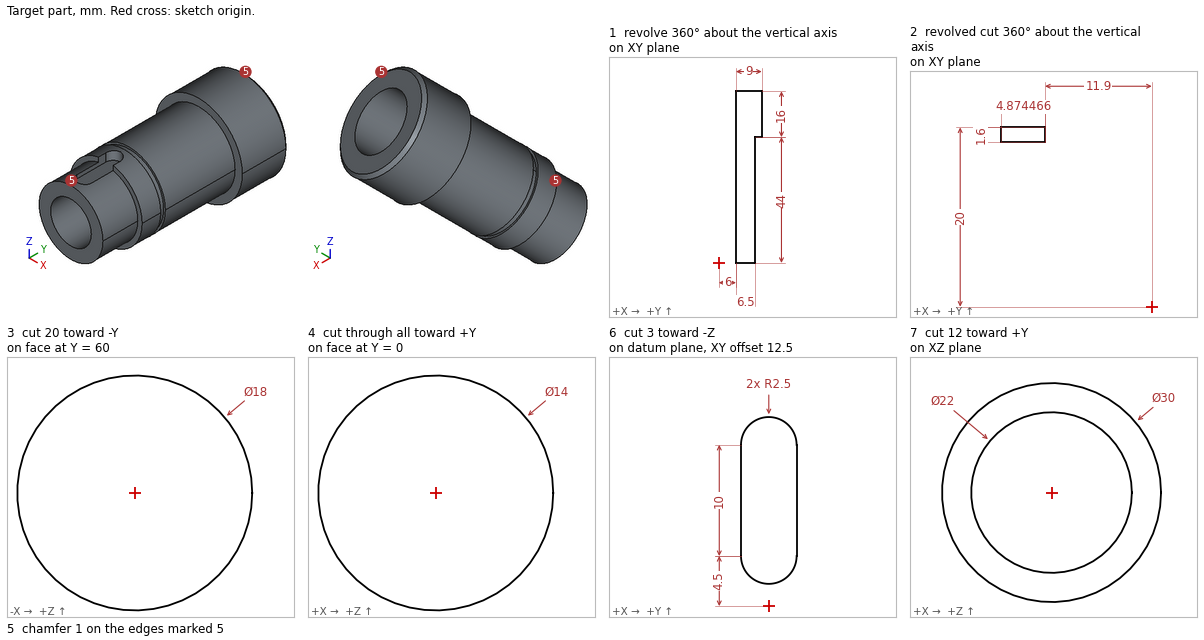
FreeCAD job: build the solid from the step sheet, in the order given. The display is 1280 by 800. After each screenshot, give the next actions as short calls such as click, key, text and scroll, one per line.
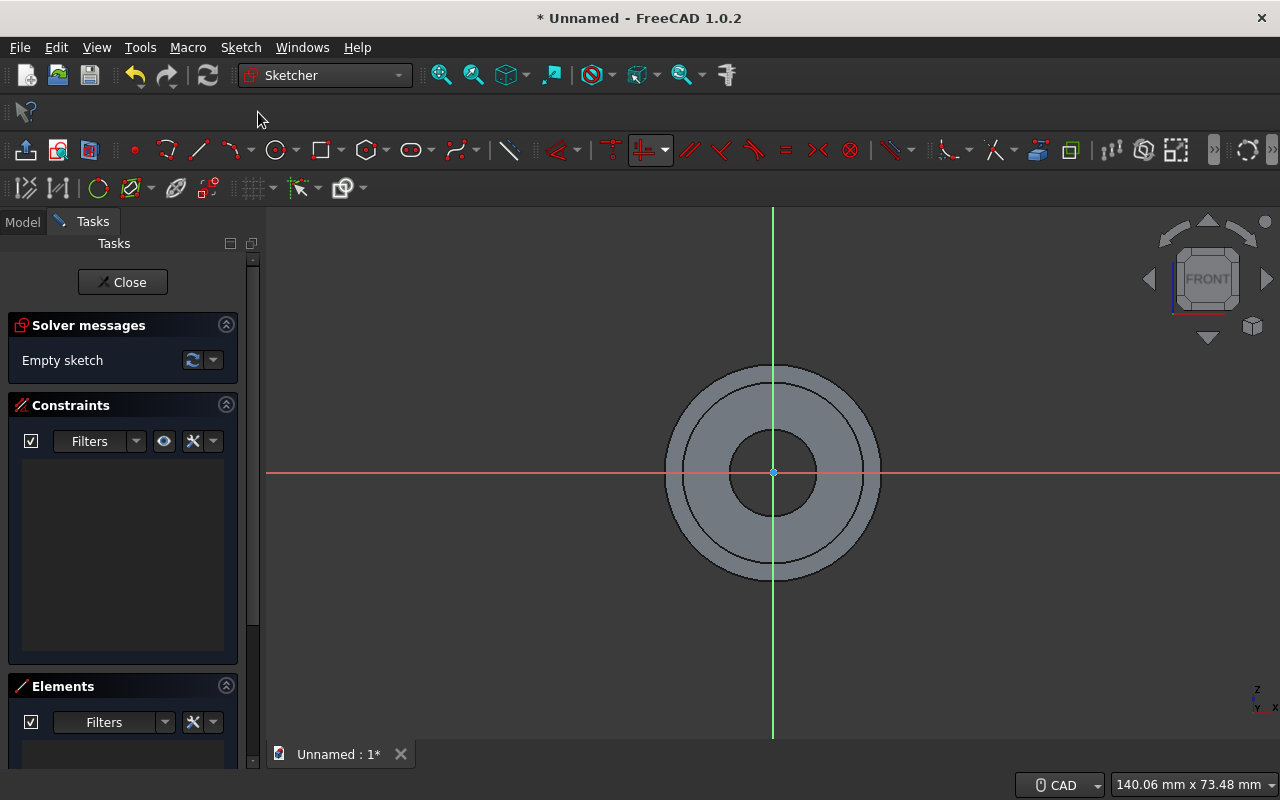
scroll(803, 473, up, 6)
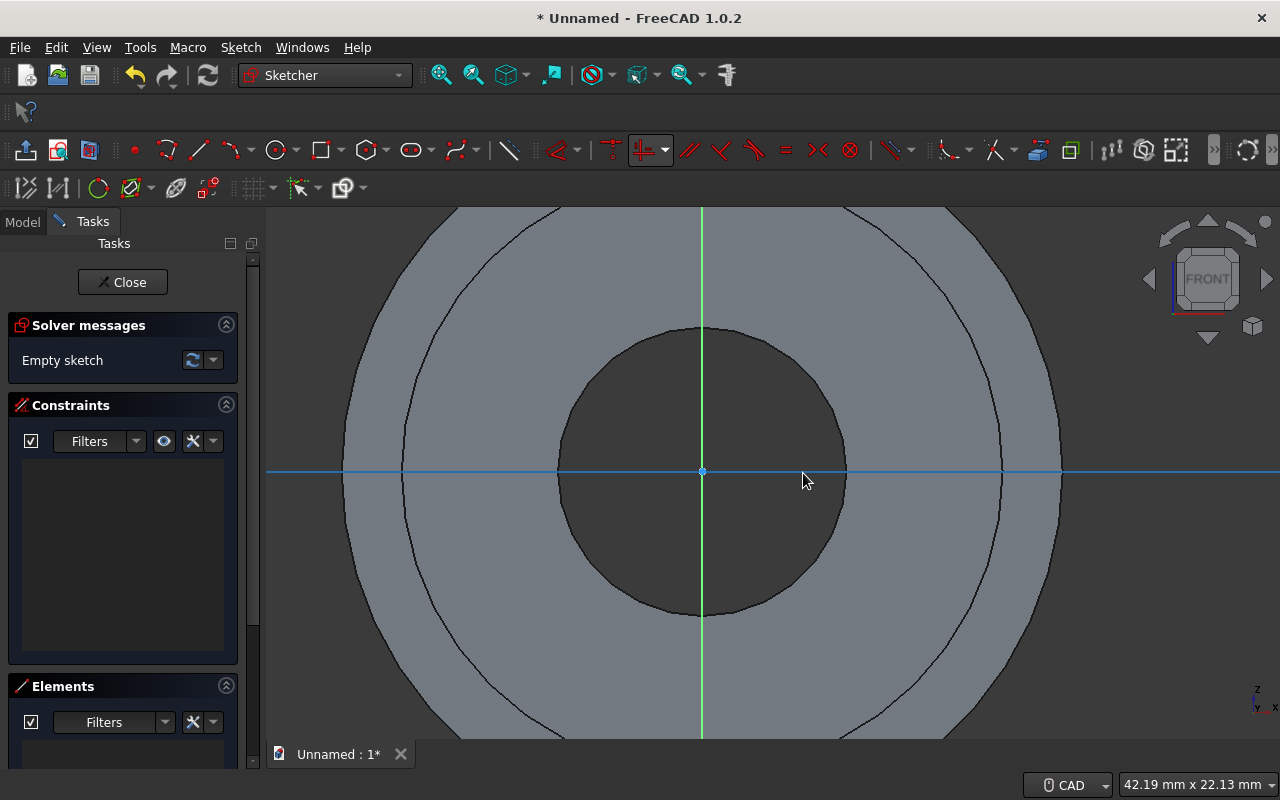
click(276, 150)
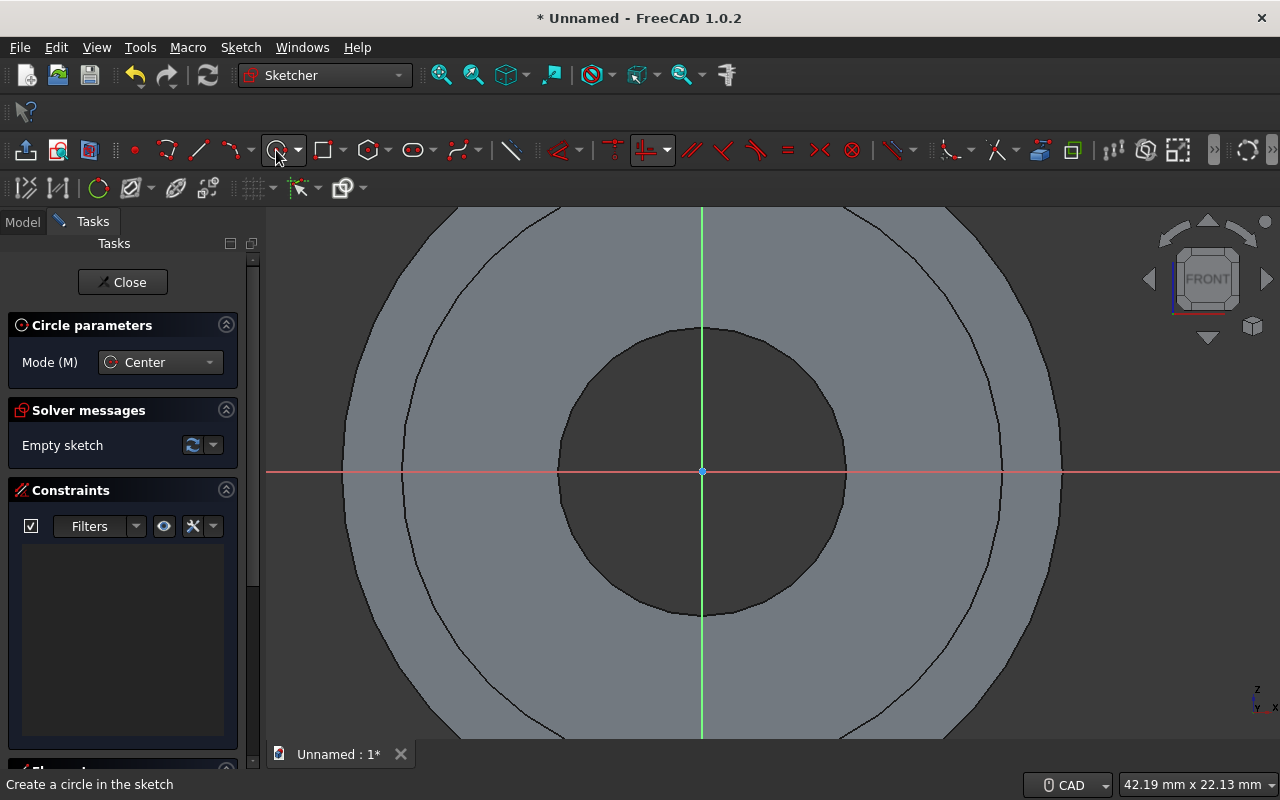
click(702, 472)
move(821, 353)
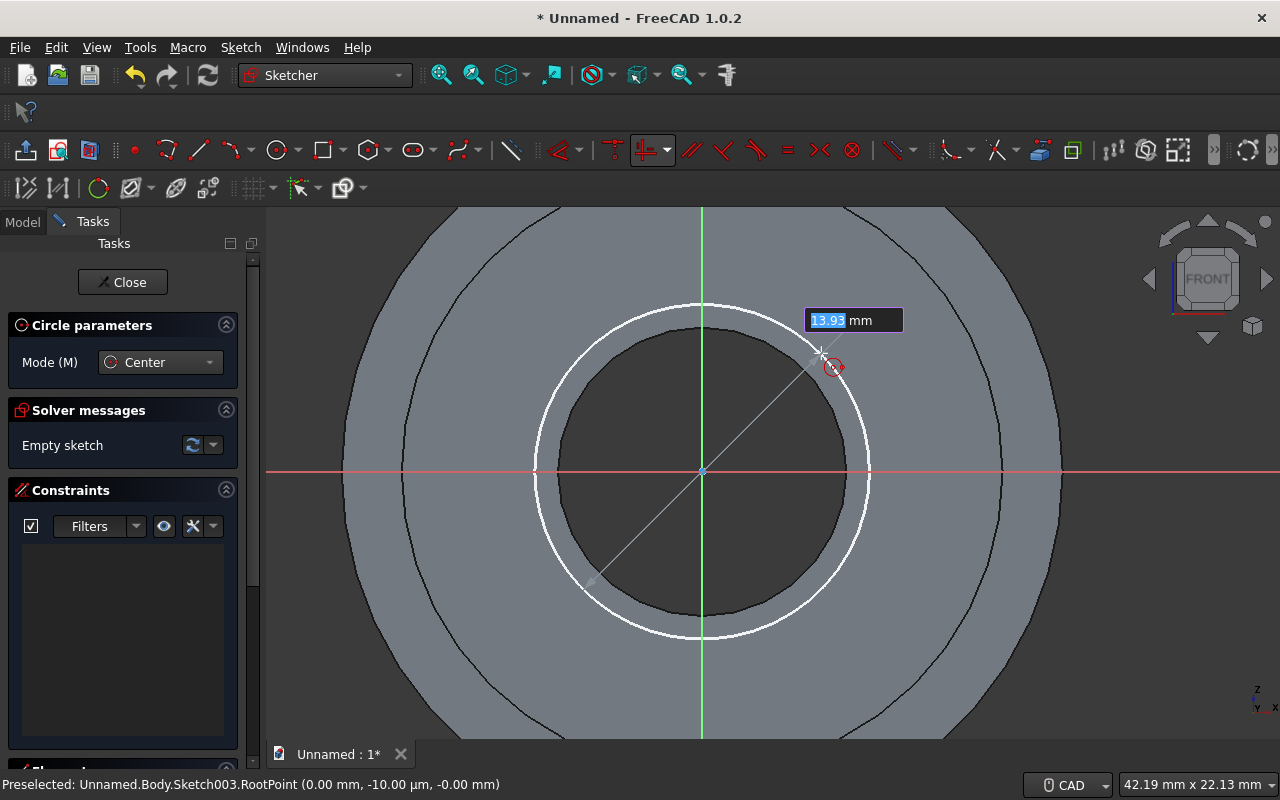
text(14)
key(Return)
key(Escape)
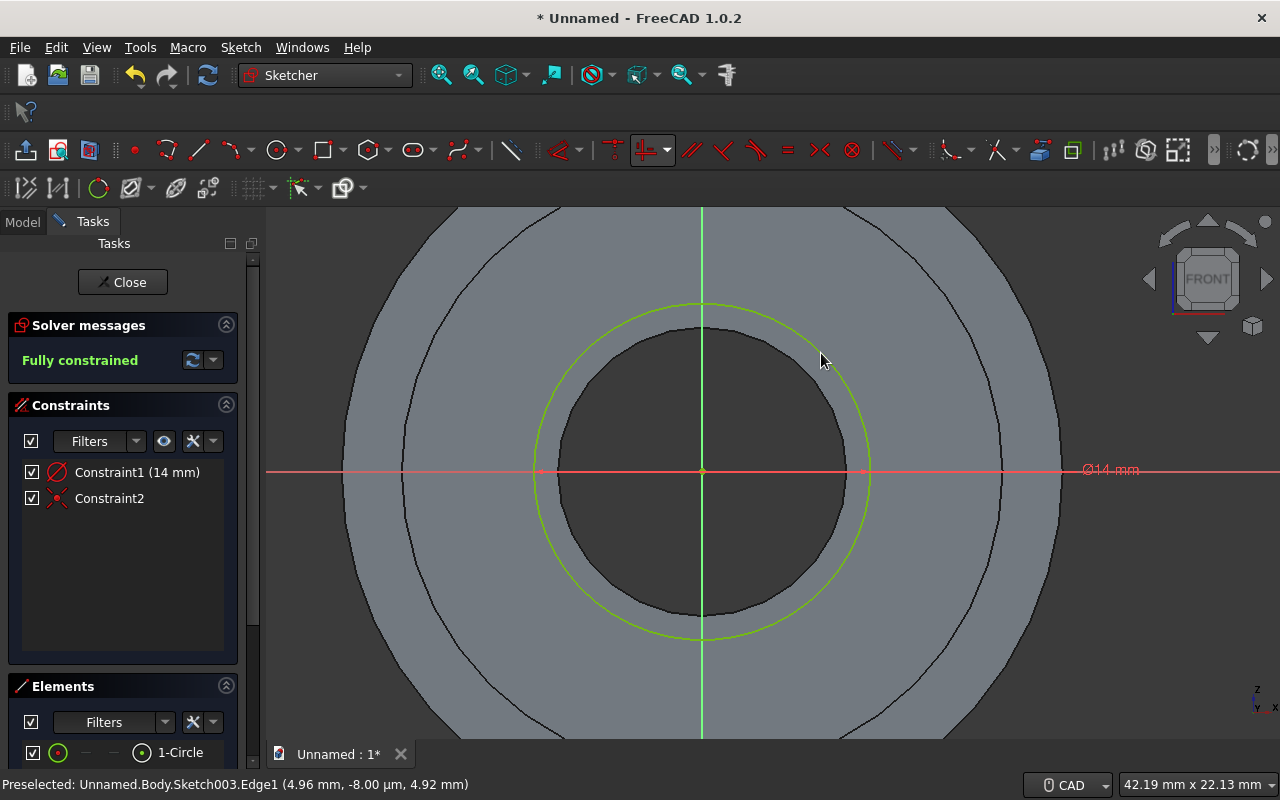
click(123, 282)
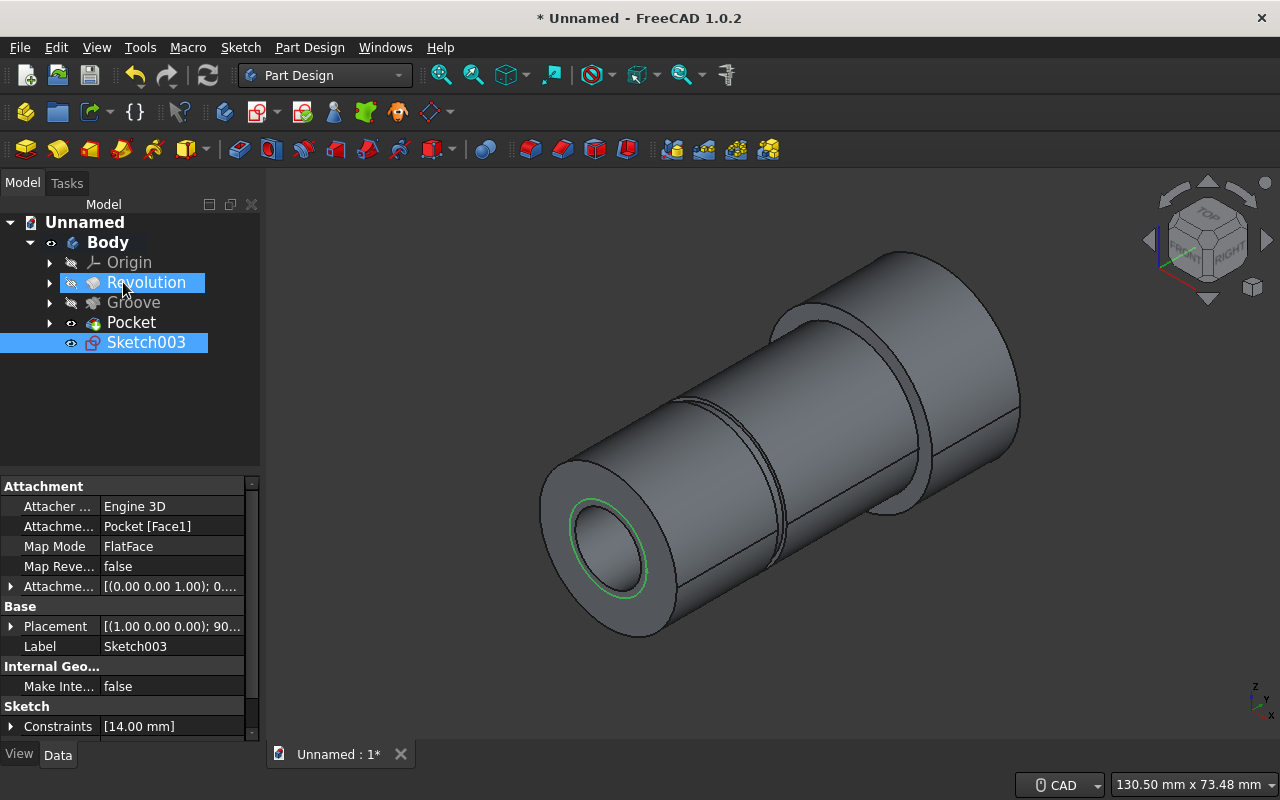
click(240, 150)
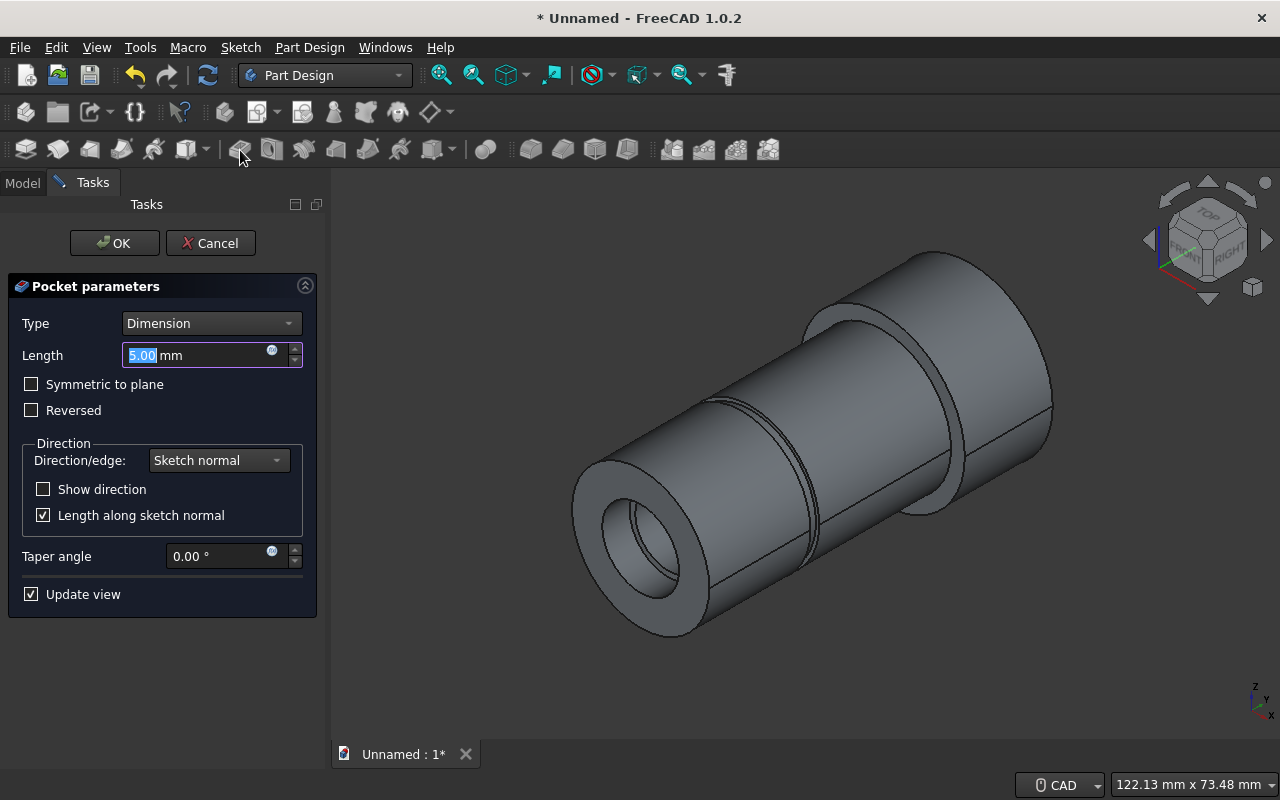
click(212, 324)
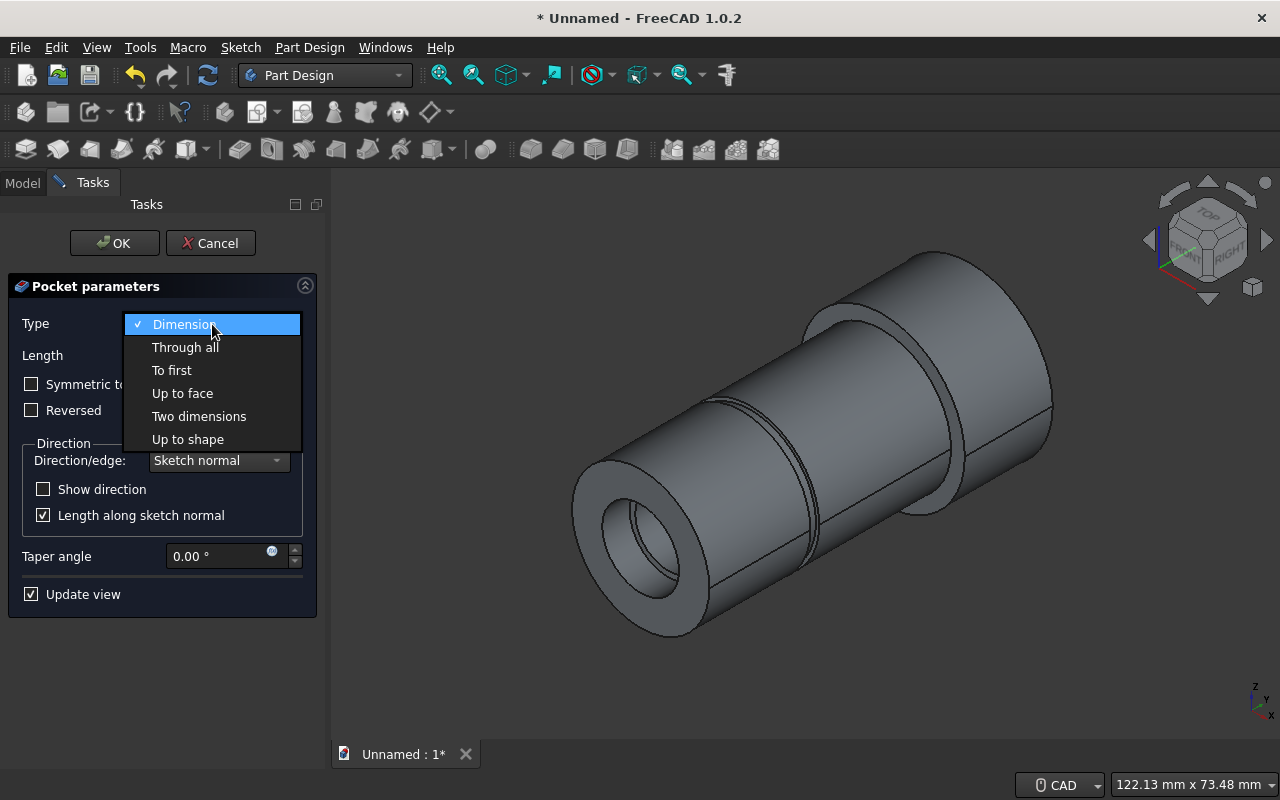
click(212, 348)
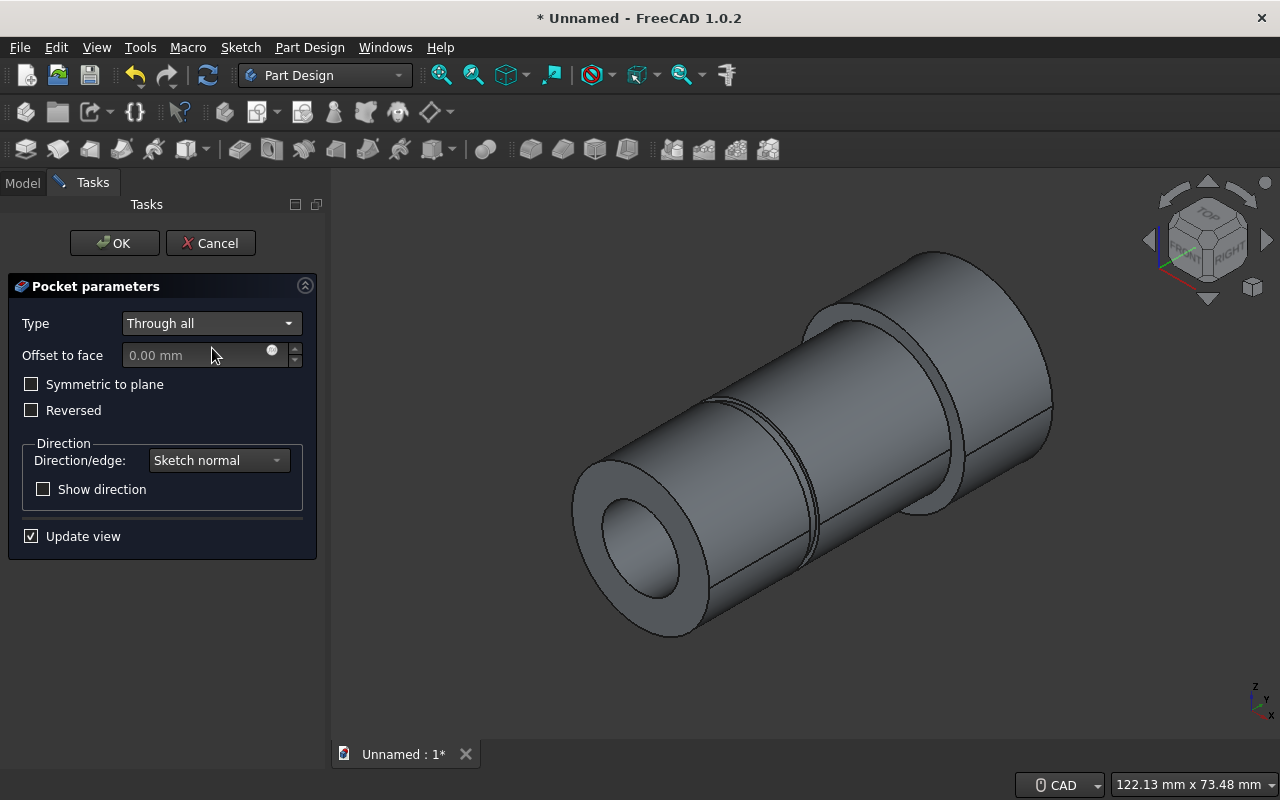
click(115, 243)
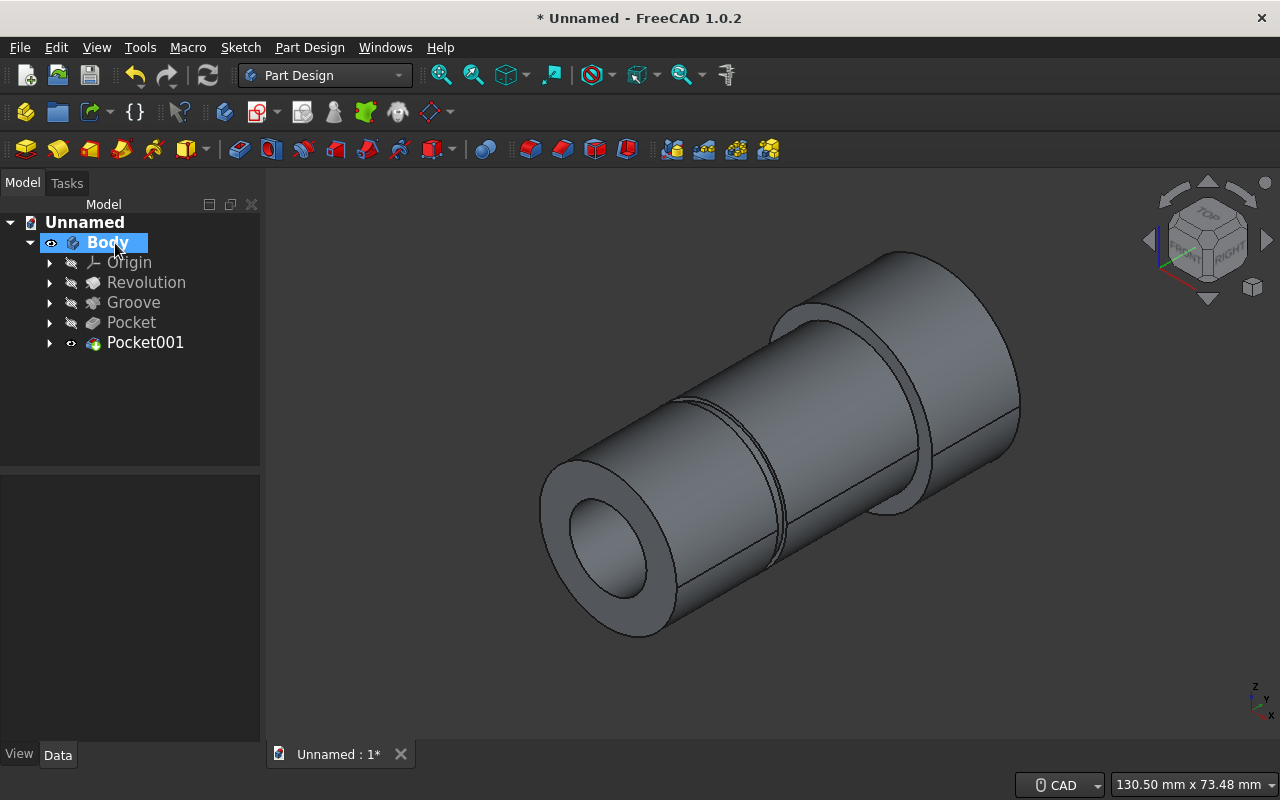
click(587, 460)